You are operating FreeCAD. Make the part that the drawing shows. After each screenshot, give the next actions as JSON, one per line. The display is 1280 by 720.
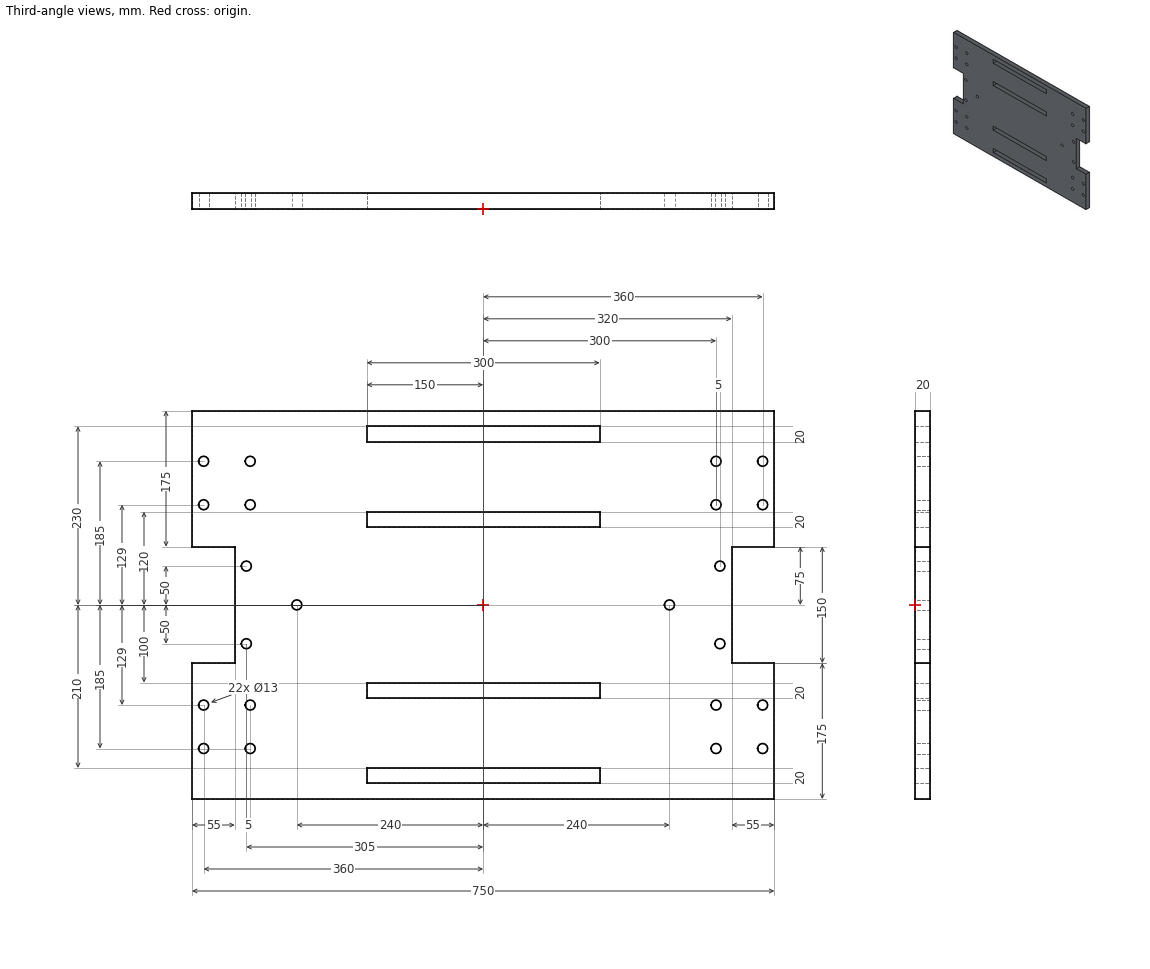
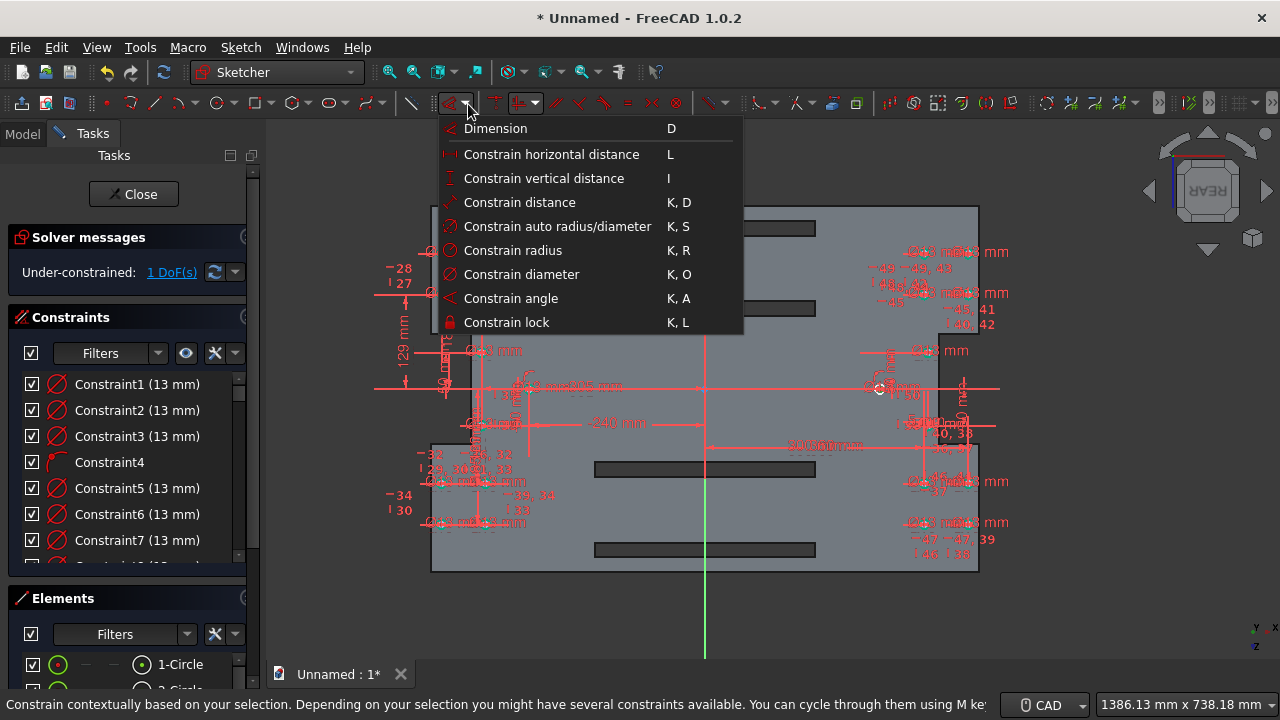
{"action": "left_click", "coordinate": [591, 154]}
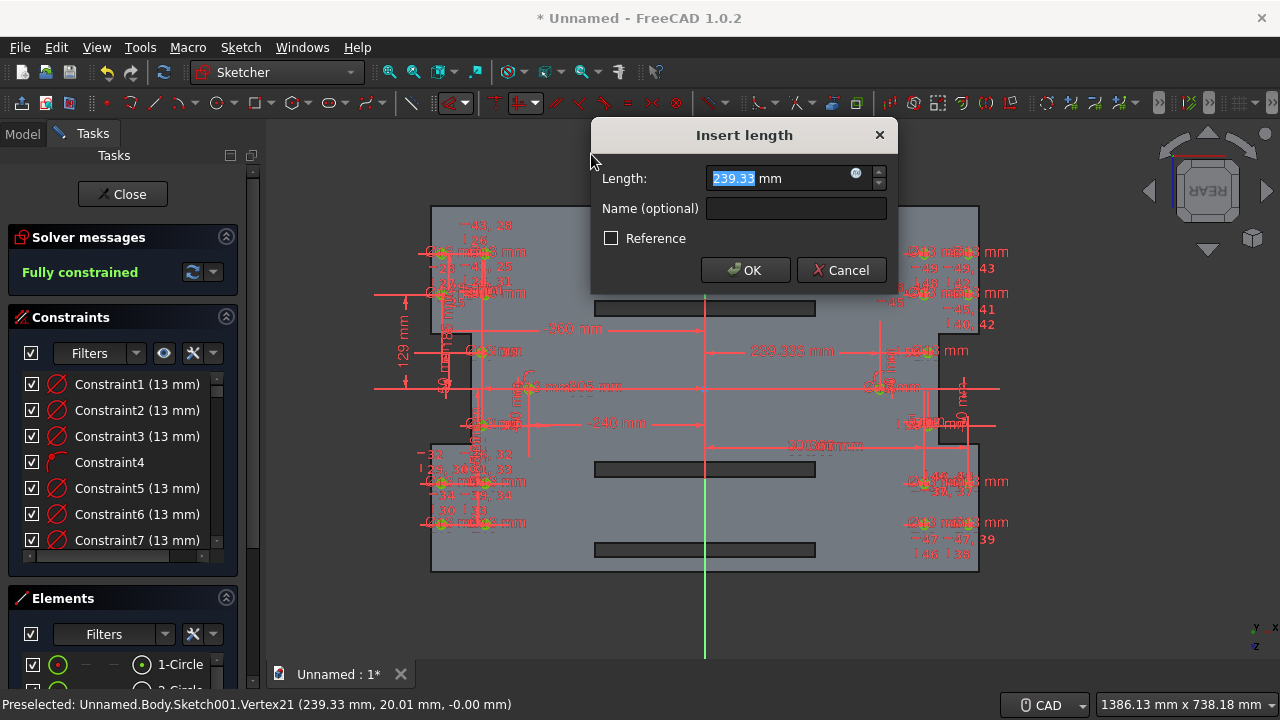
{"action": "type", "text": "240"}
{"action": "key", "text": "Return"}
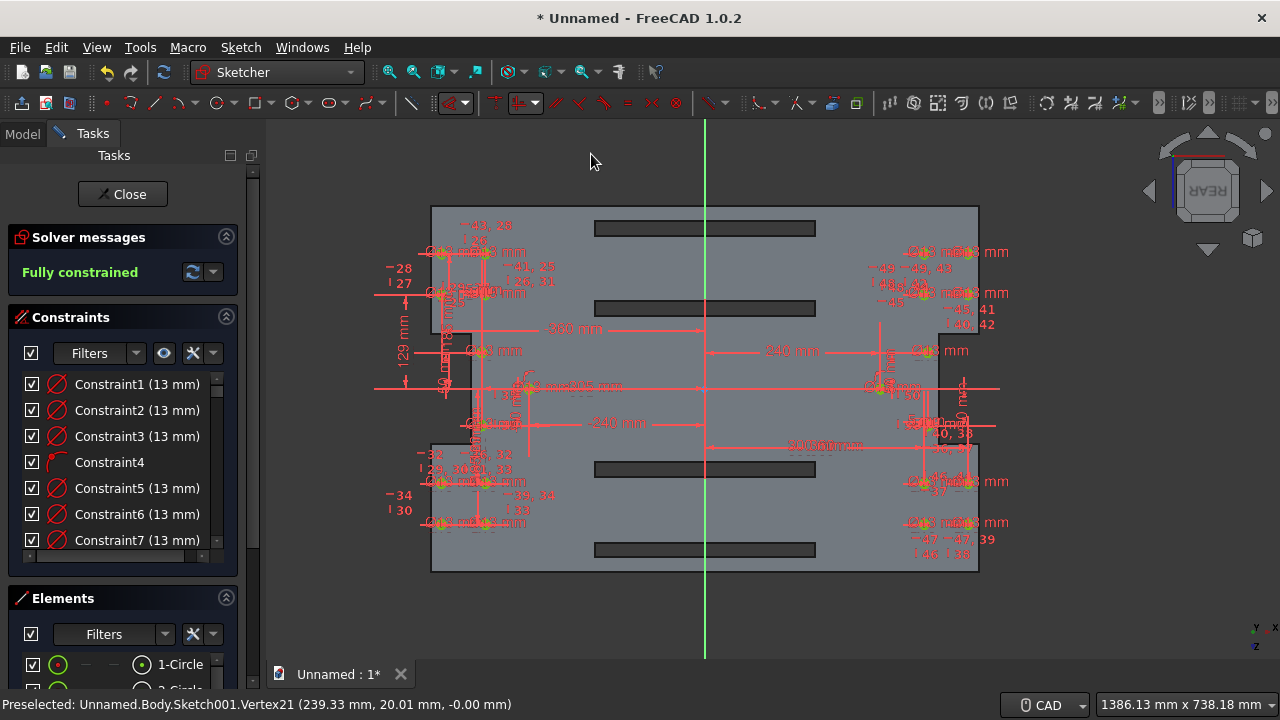
{"action": "left_click", "coordinate": [123, 194]}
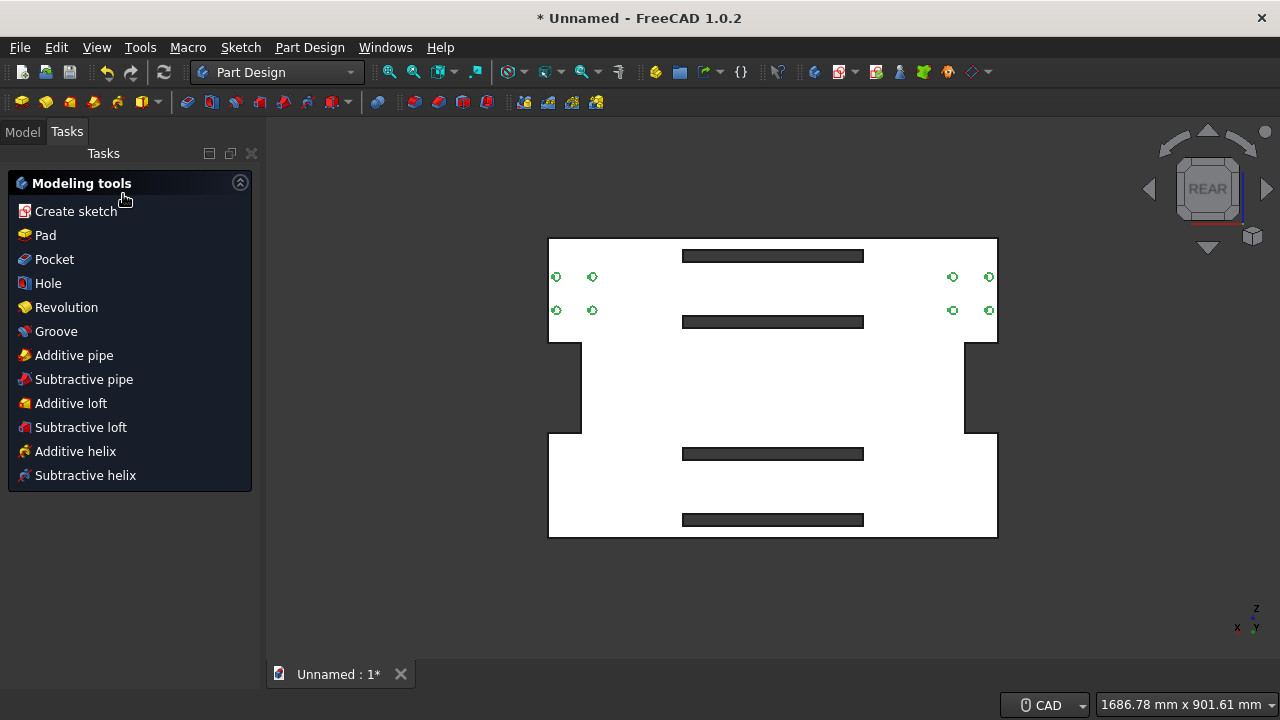
{"action": "left_click", "coordinate": [188, 102]}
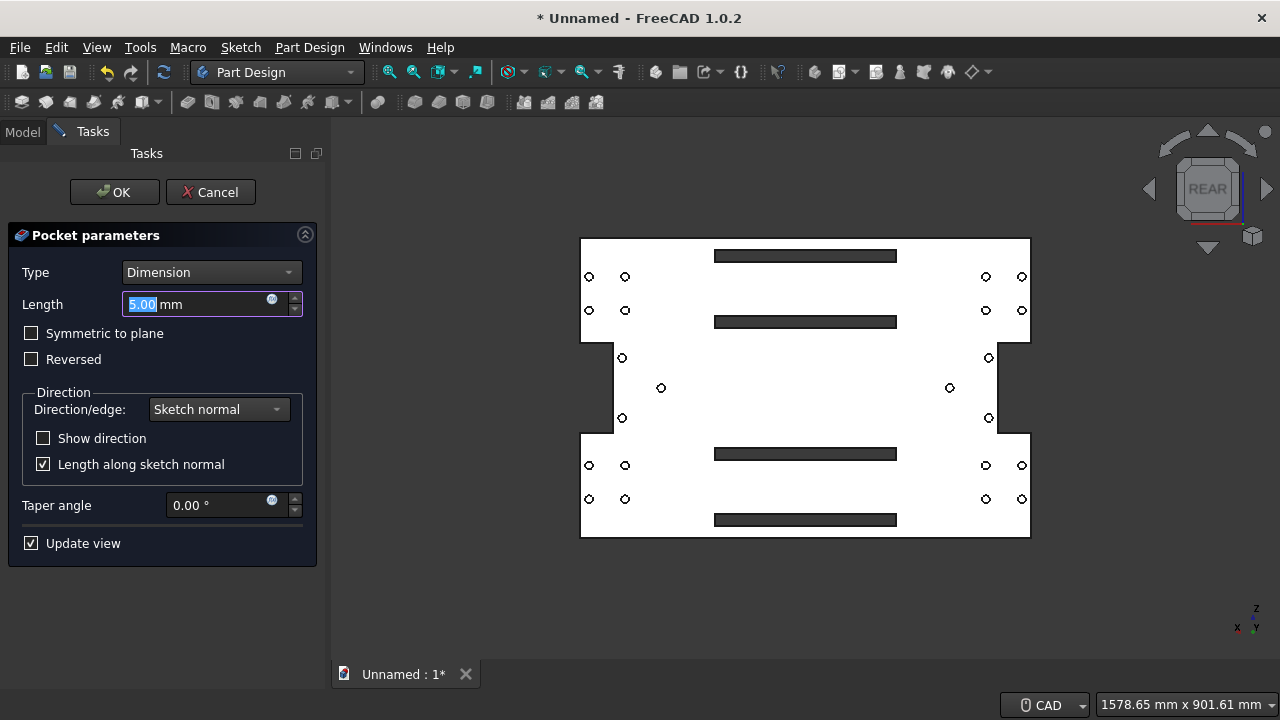
{"action": "left_click", "coordinate": [212, 272]}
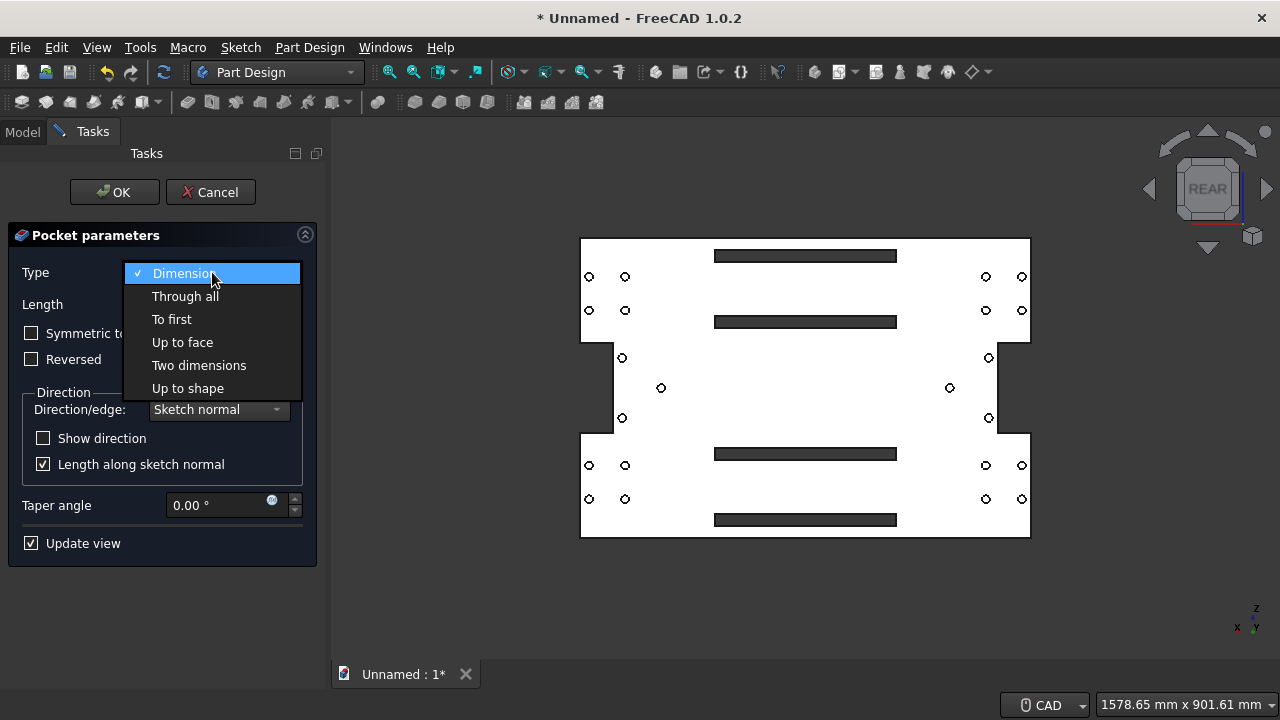
{"action": "left_click", "coordinate": [212, 296]}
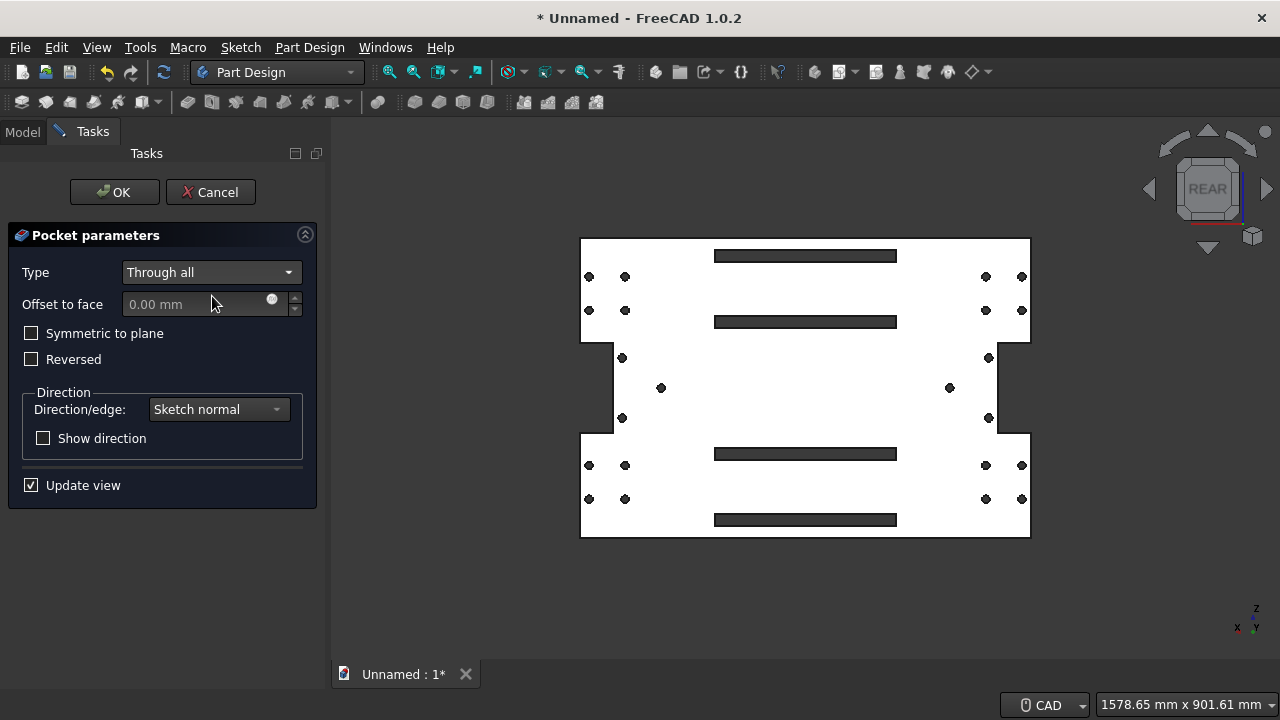
{"action": "left_click", "coordinate": [115, 192]}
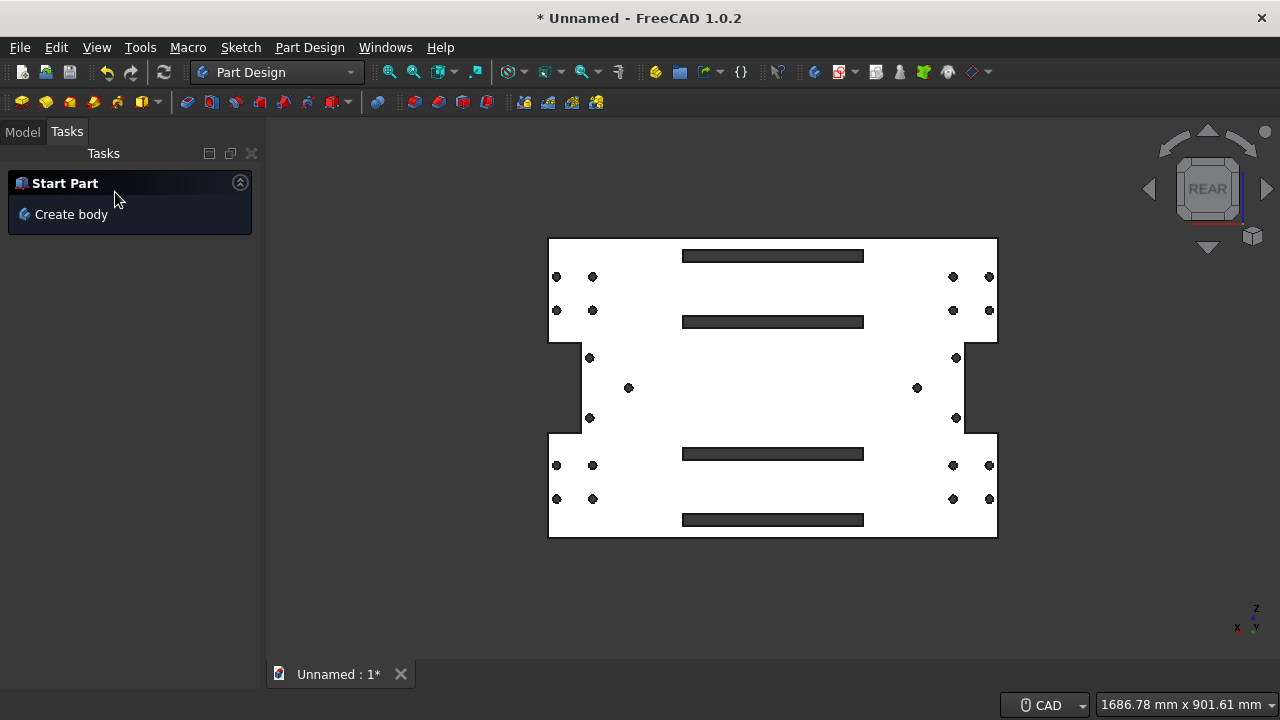
{"action": "key", "text": "0"}